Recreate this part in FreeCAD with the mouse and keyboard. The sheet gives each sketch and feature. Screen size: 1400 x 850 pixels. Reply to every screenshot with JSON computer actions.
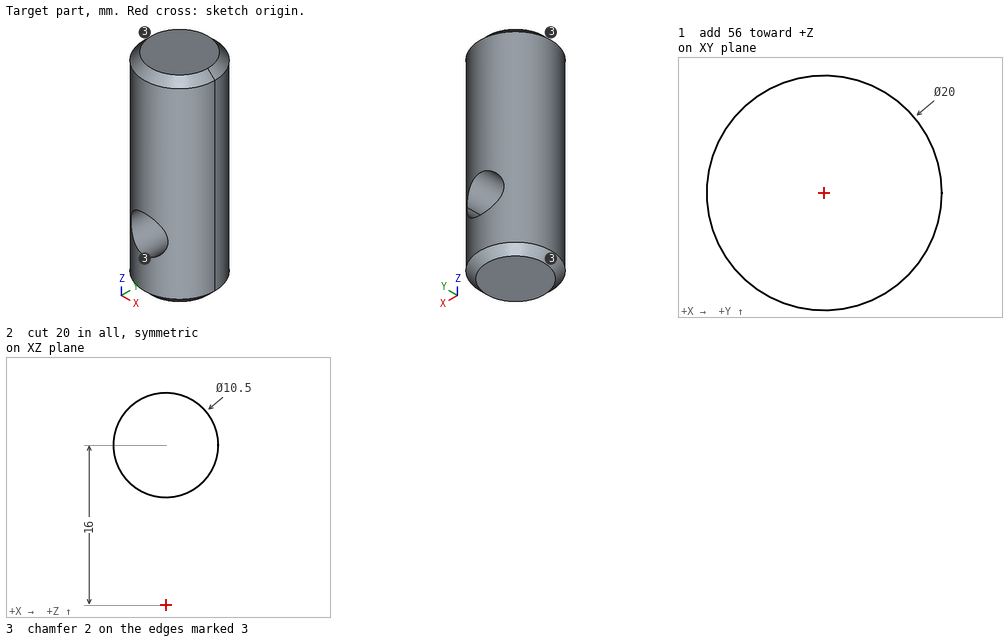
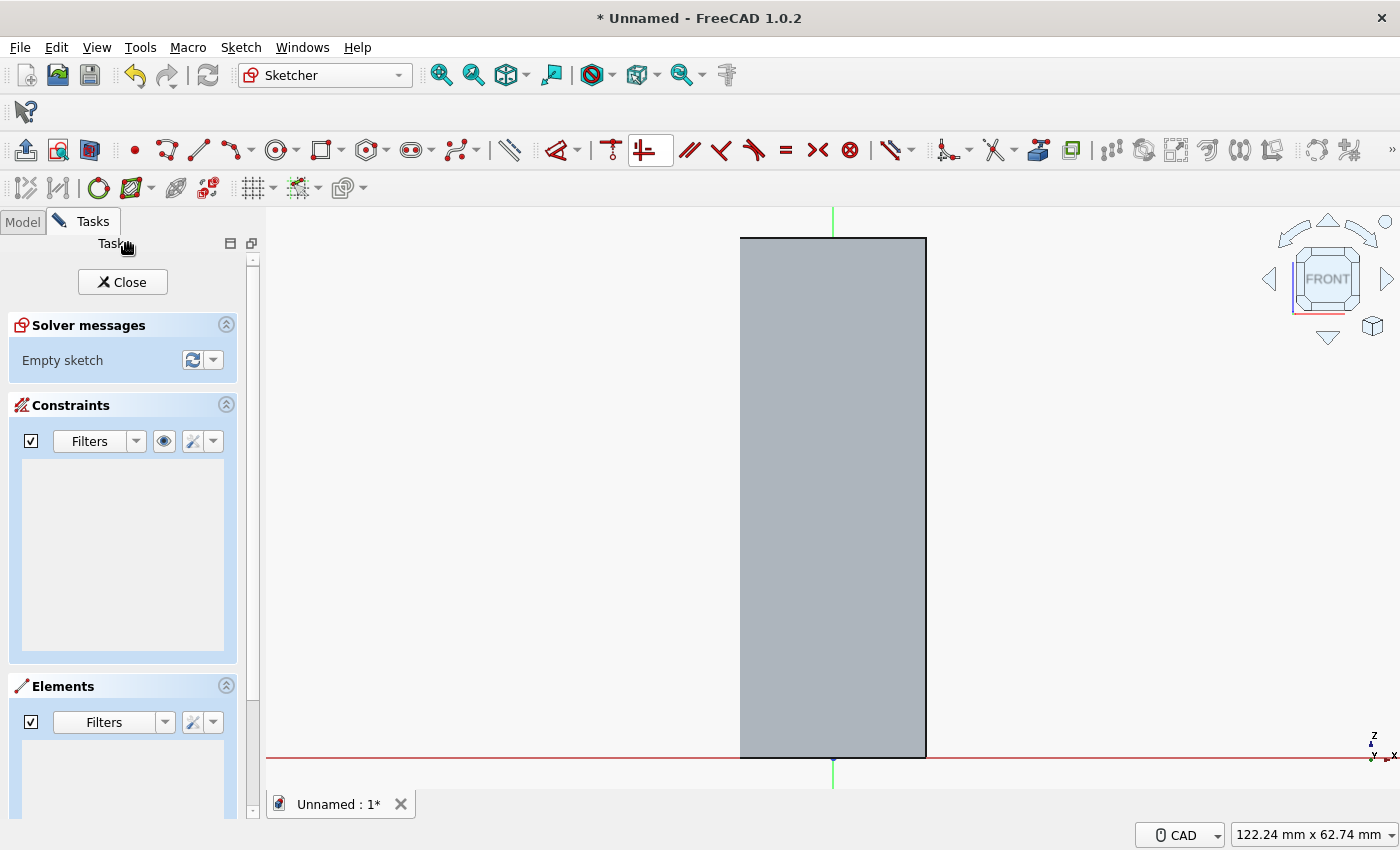
{"action": "left_click", "coordinate": [90, 150]}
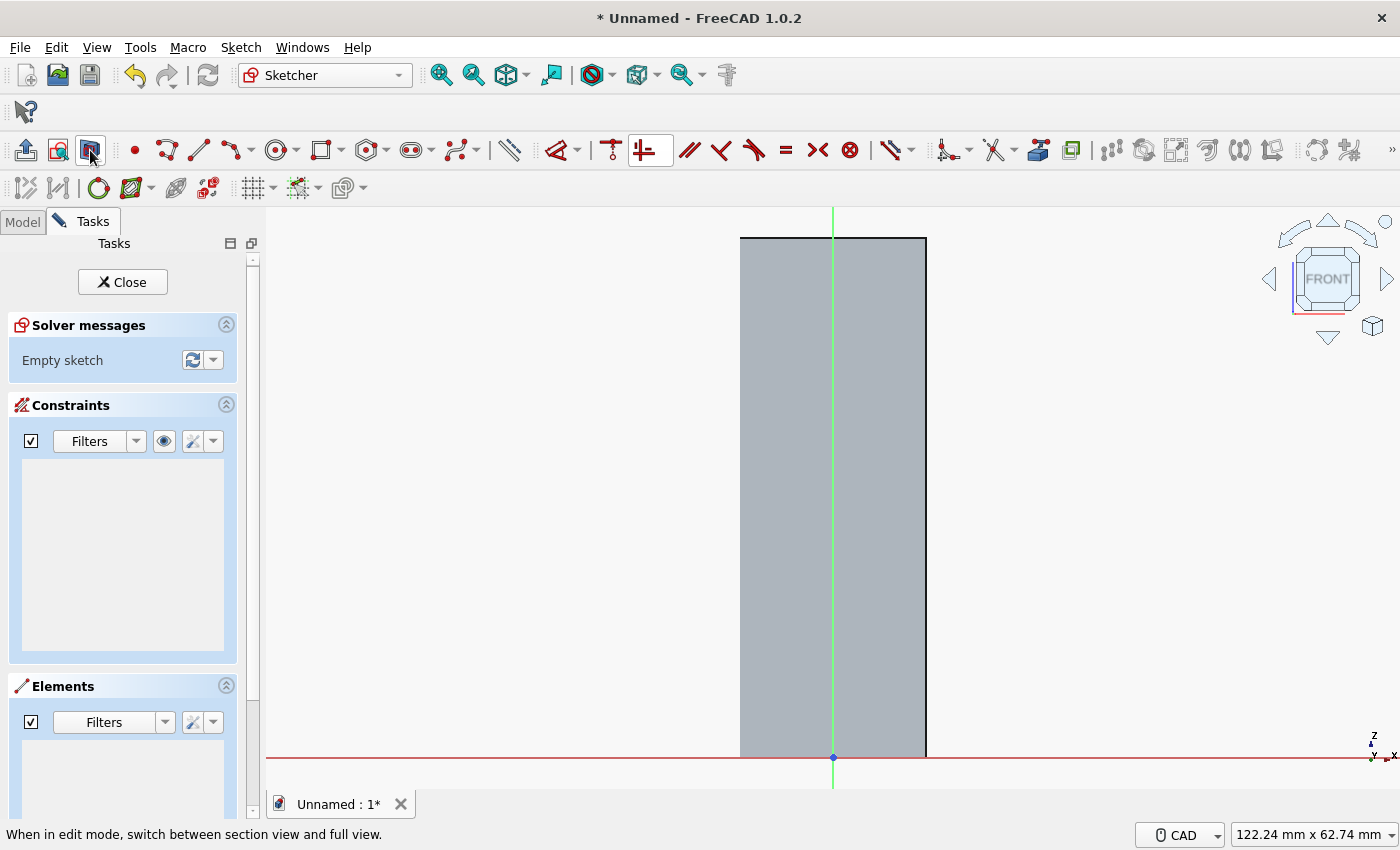
{"action": "scroll", "coordinate": [764, 498], "scroll_direction": "down", "scroll_amount": 5}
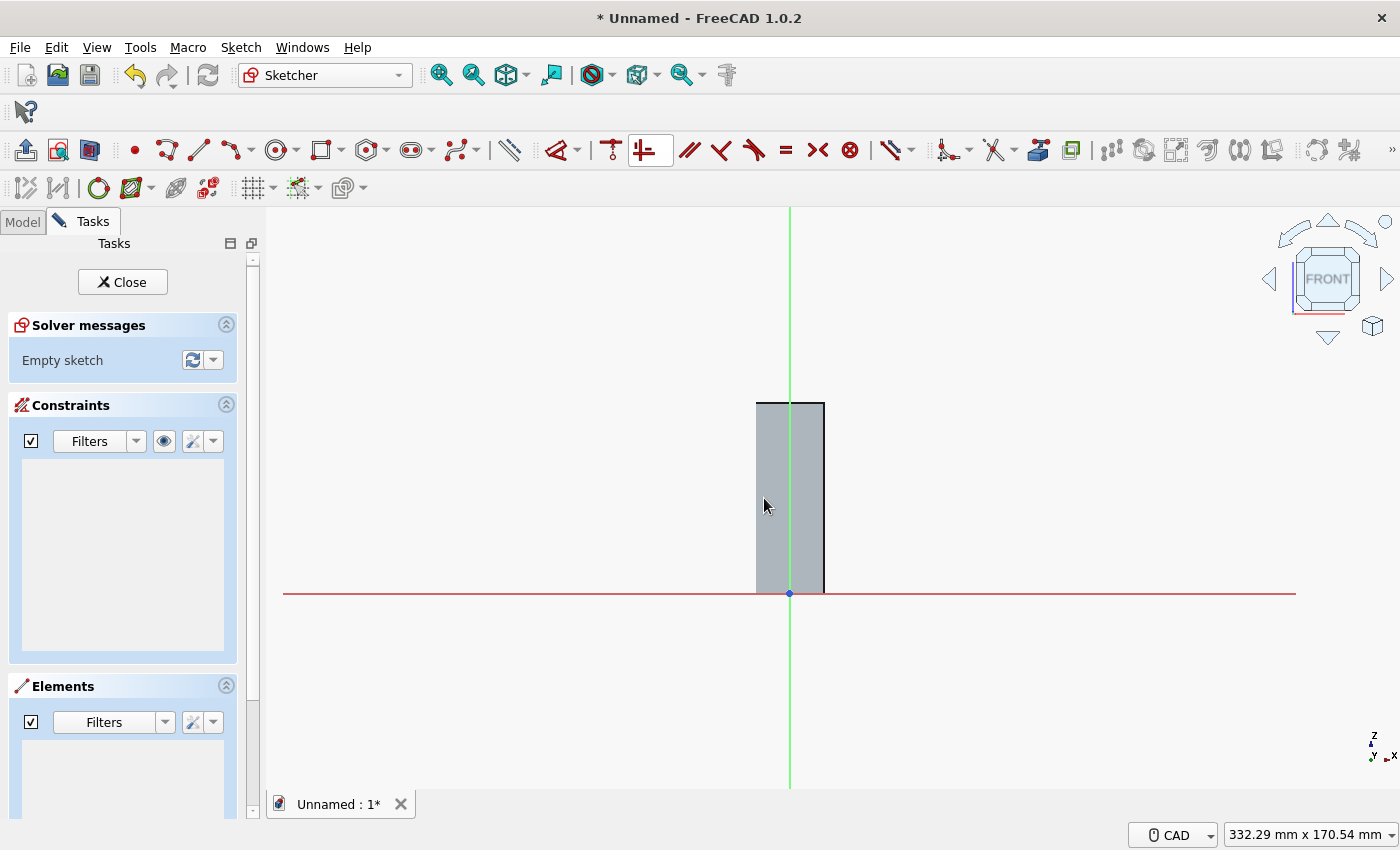
{"action": "scroll", "coordinate": [796, 573], "scroll_direction": "up", "scroll_amount": 8}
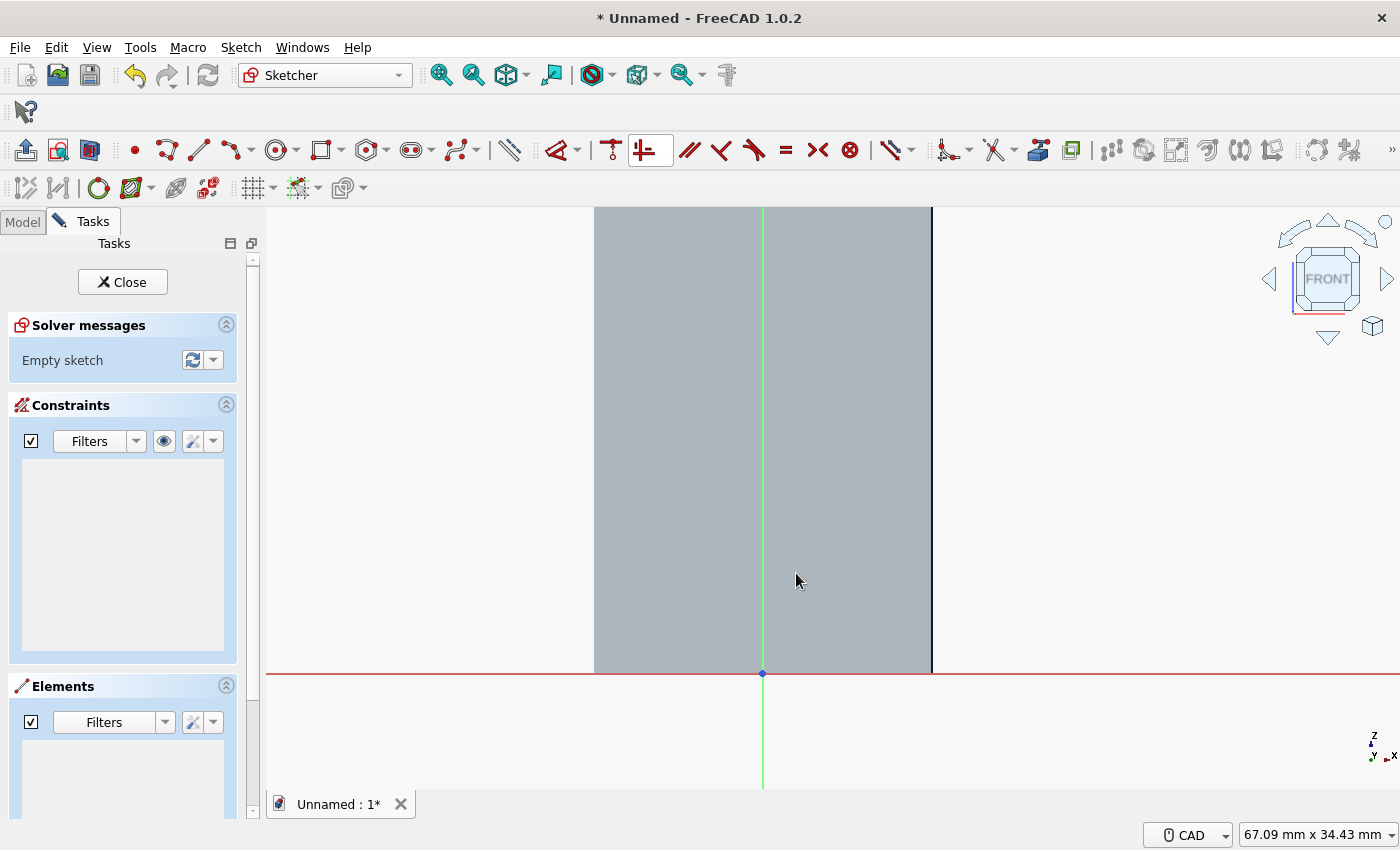
{"action": "left_click", "coordinate": [276, 150]}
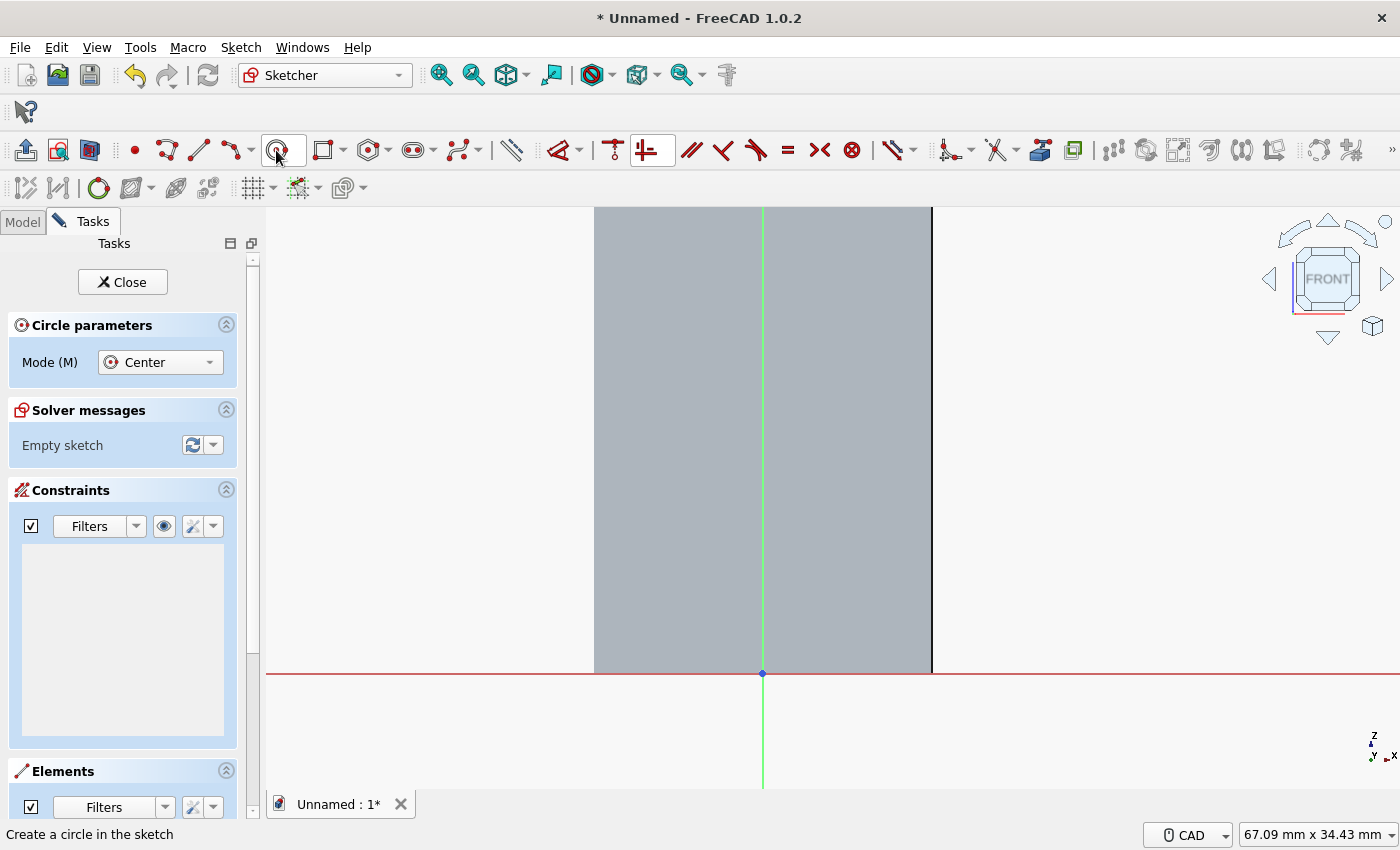
{"action": "left_click", "coordinate": [763, 403]}
{"action": "left_click", "coordinate": [826, 341]}
{"action": "key", "text": "Escape"}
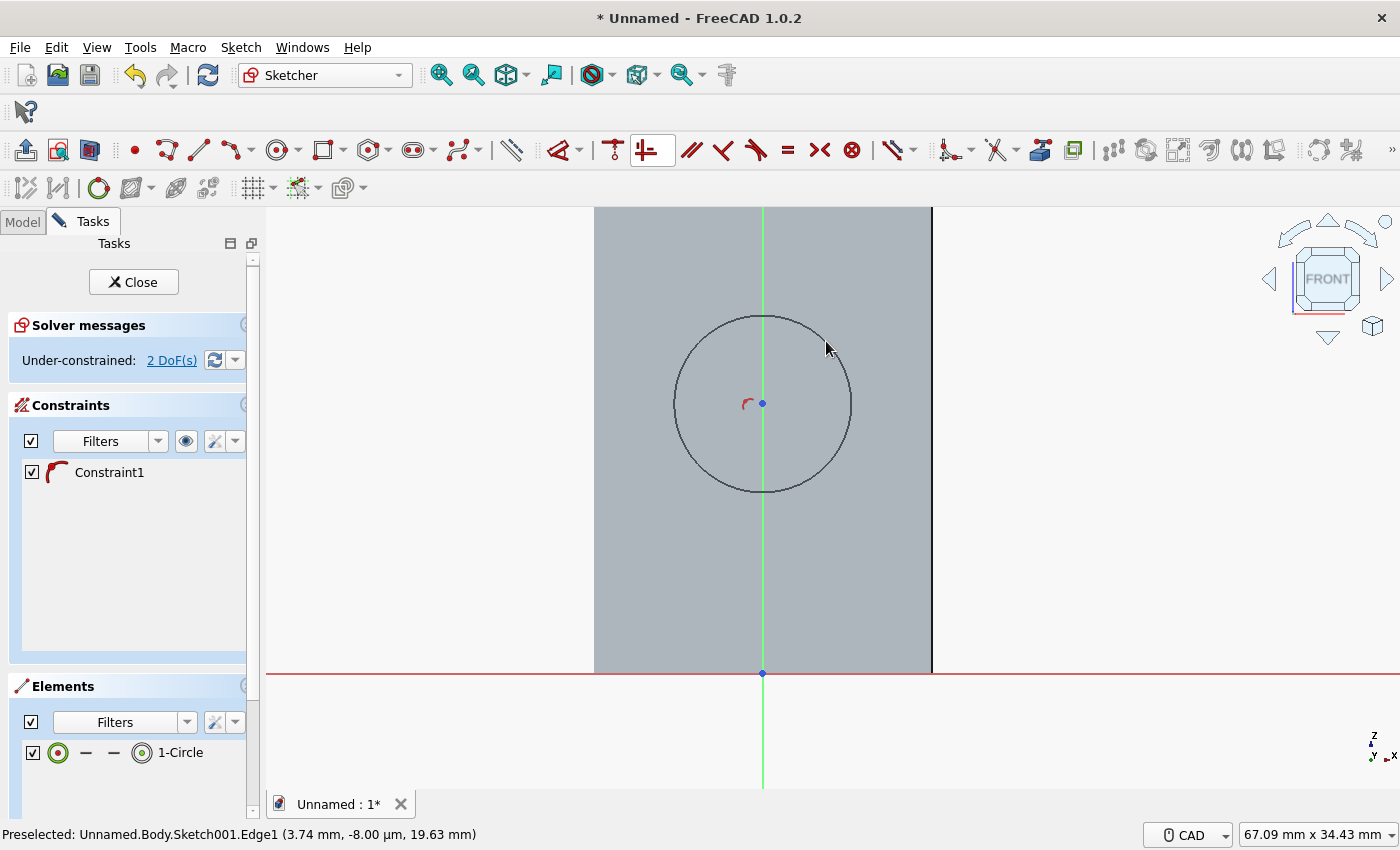
{"action": "left_click", "coordinate": [558, 150]}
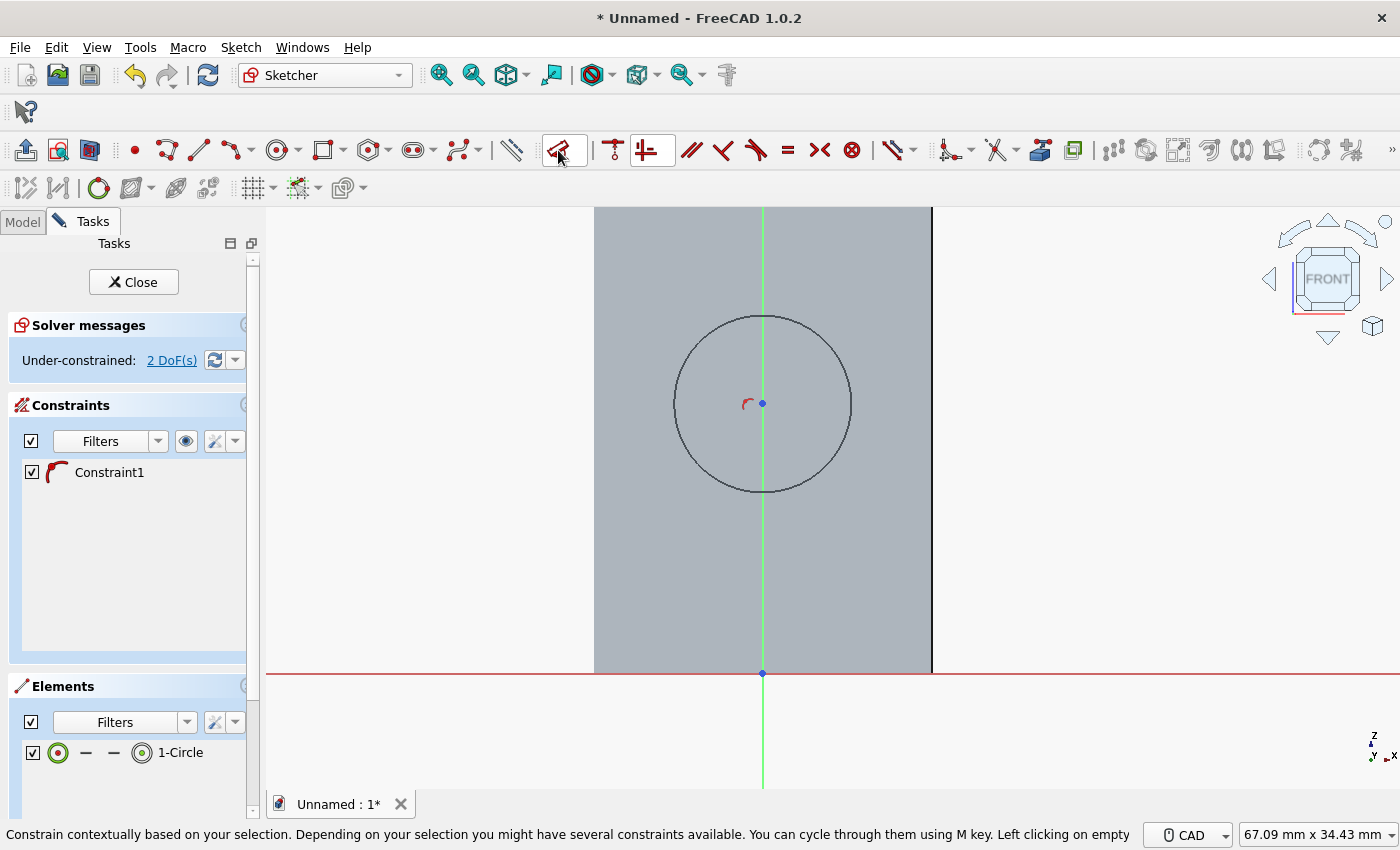
{"action": "left_click", "coordinate": [825, 341]}
{"action": "left_click", "coordinate": [847, 318]}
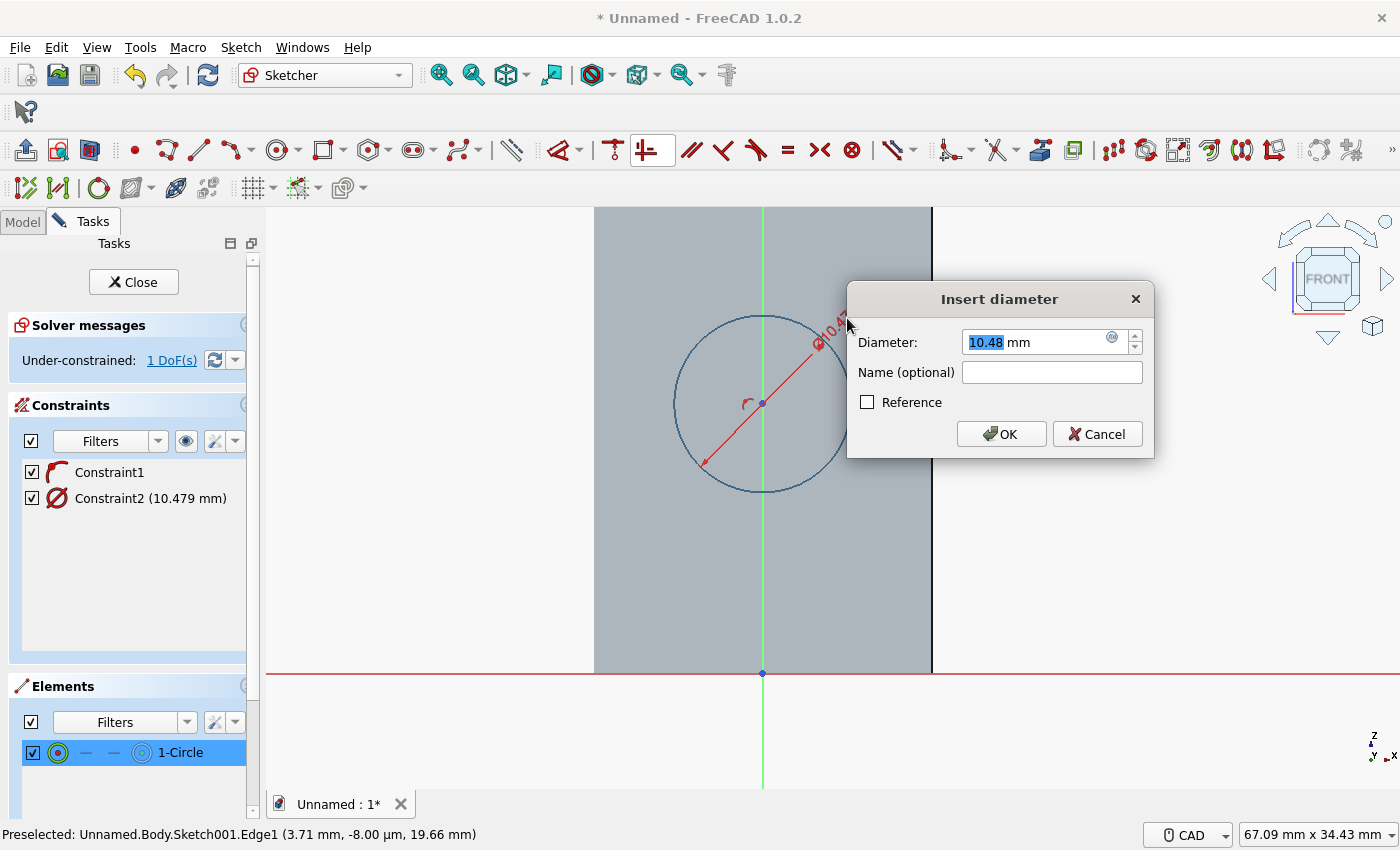
{"action": "type", "text": "10.5"}
{"action": "key", "text": "Return"}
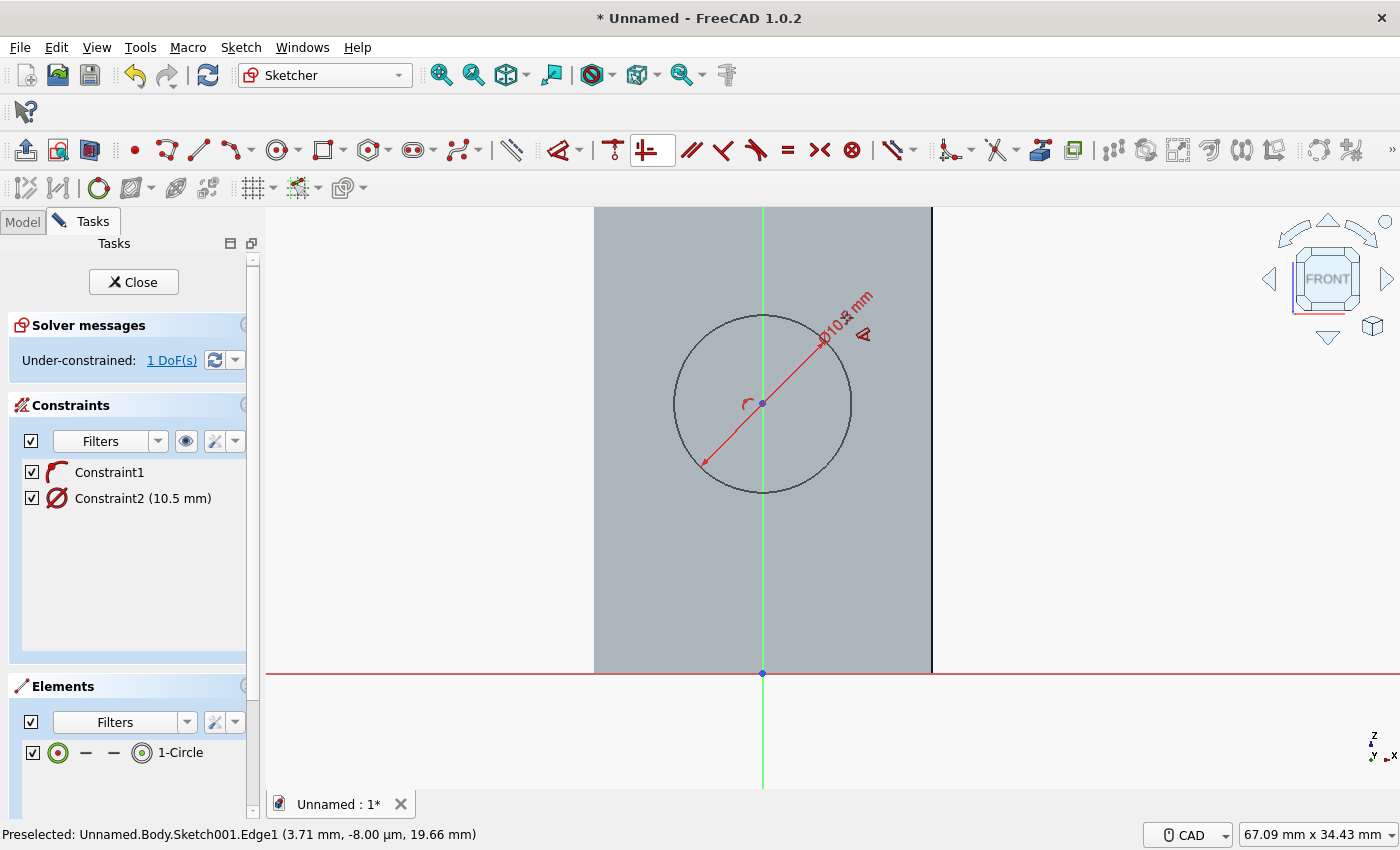
{"action": "left_click", "coordinate": [763, 404]}
{"action": "left_click", "coordinate": [797, 539]}